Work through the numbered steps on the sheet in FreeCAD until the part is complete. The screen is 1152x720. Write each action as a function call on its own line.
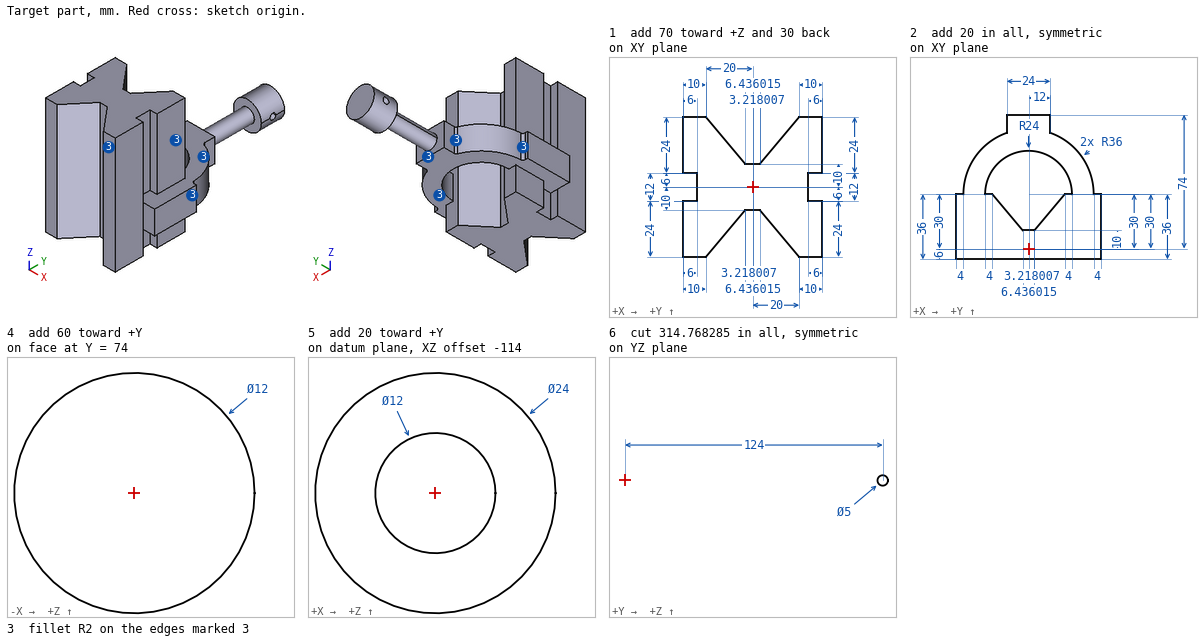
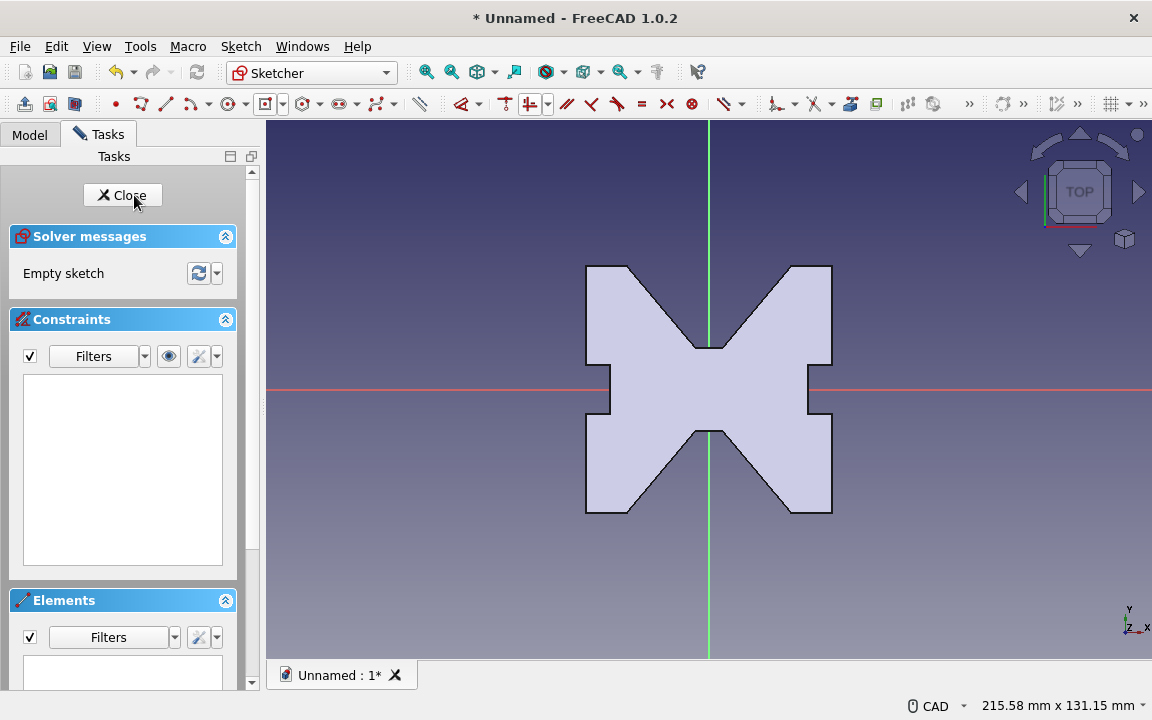
click(75, 104)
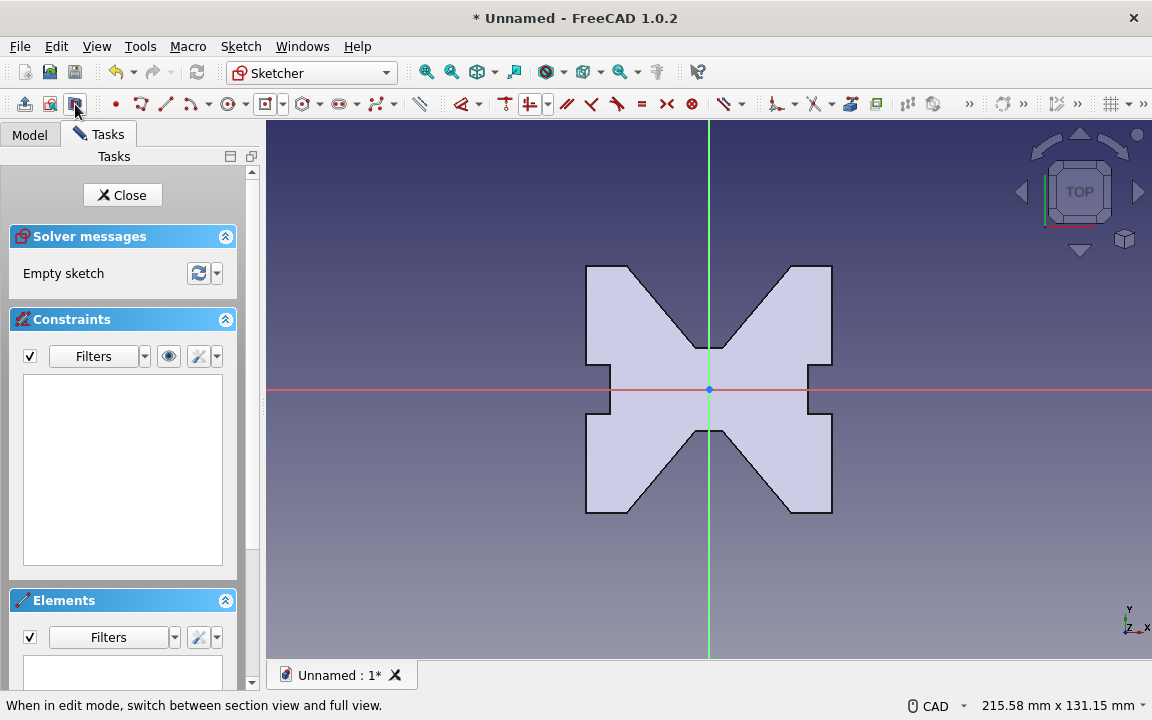
scroll(331, 631, down, 1)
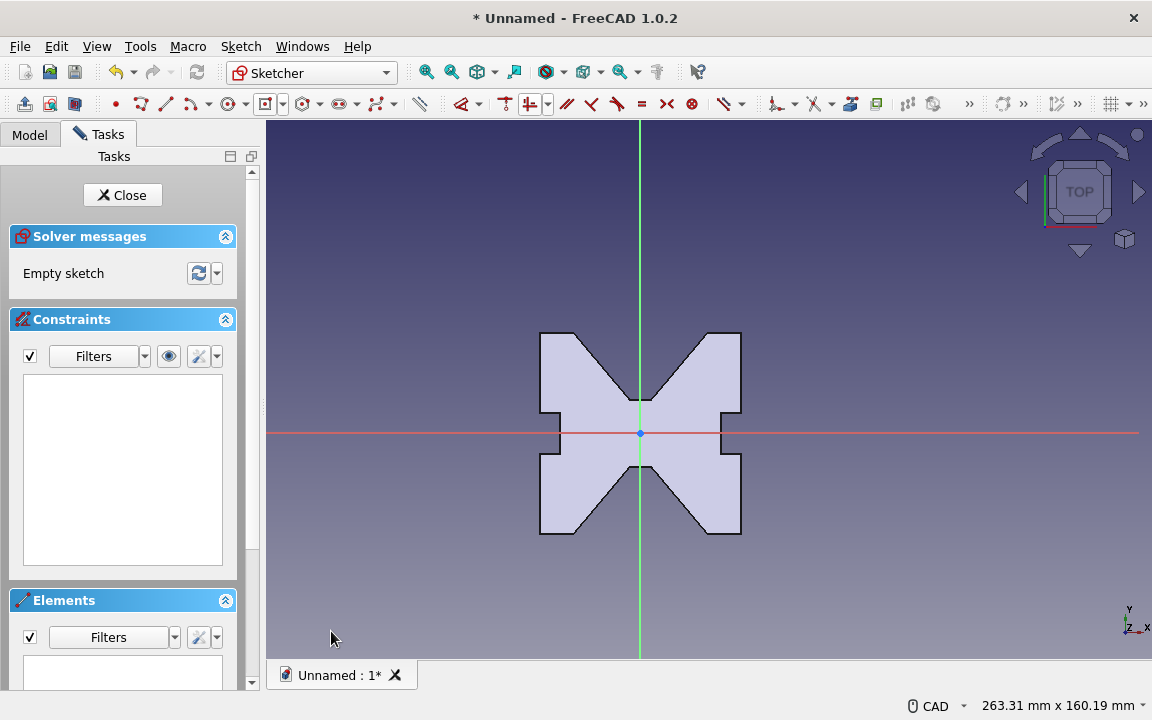
click(141, 104)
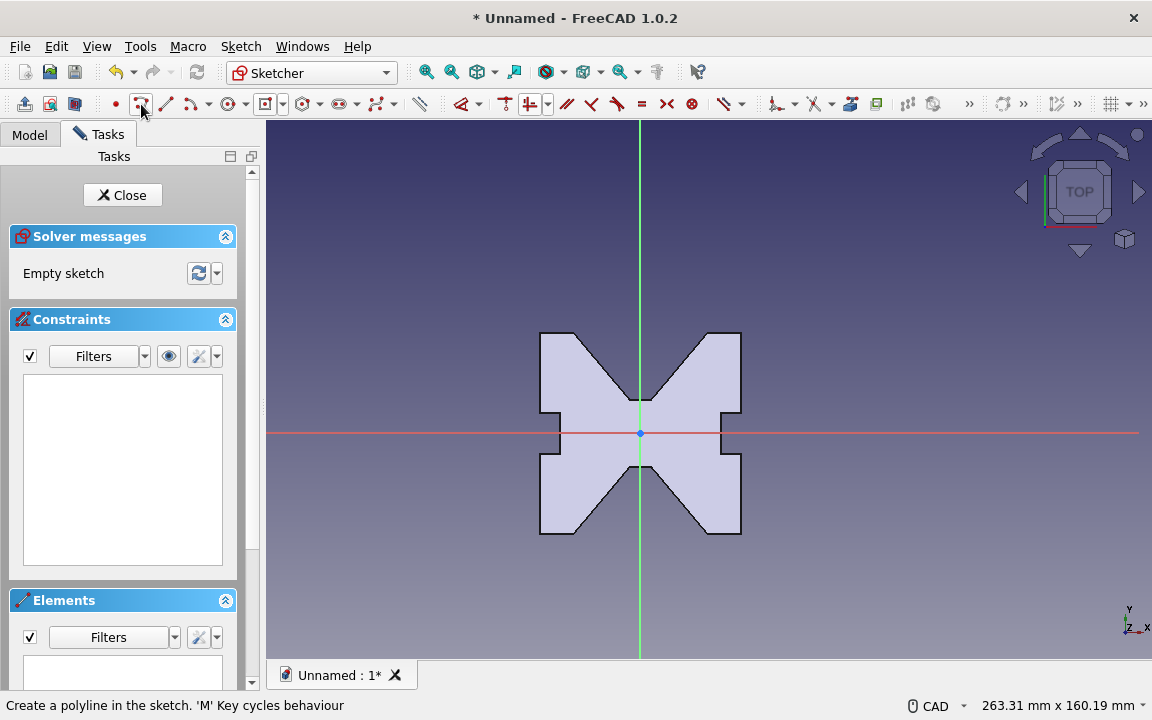
click(681, 218)
click(681, 184)
click(600, 184)
click(600, 218)
right_click(600, 218)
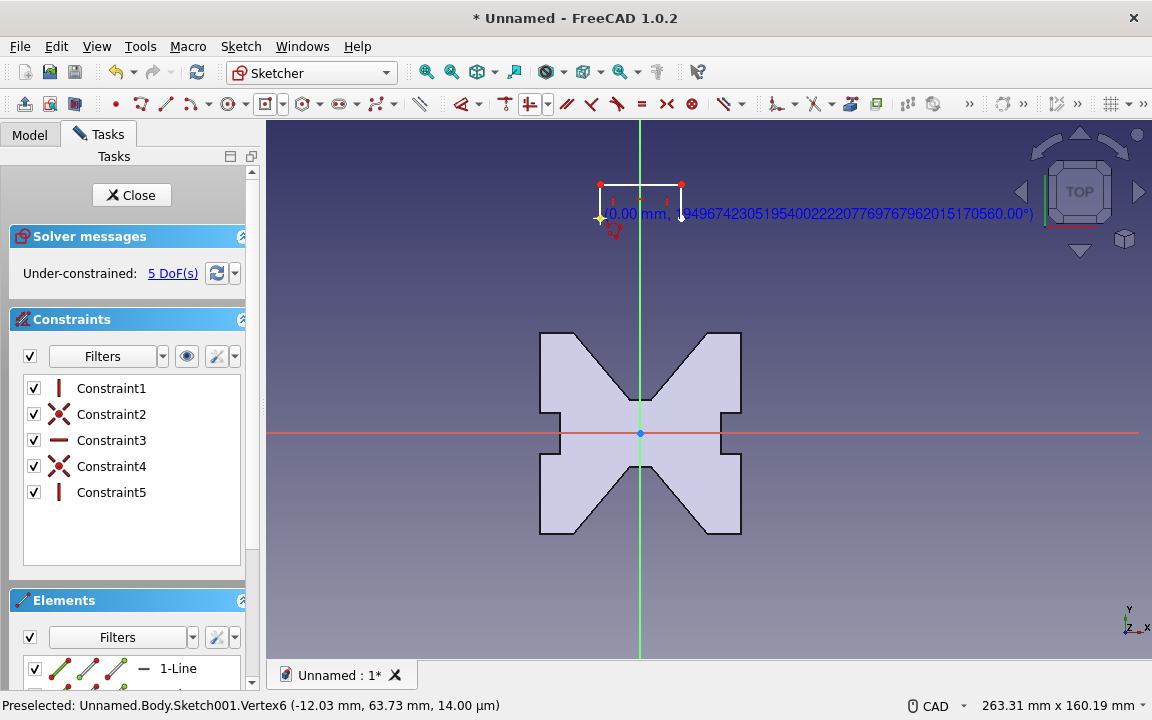
click(519, 333)
click(506, 333)
click(506, 454)
click(775, 454)
click(775, 333)
click(762, 333)
right_click(762, 333)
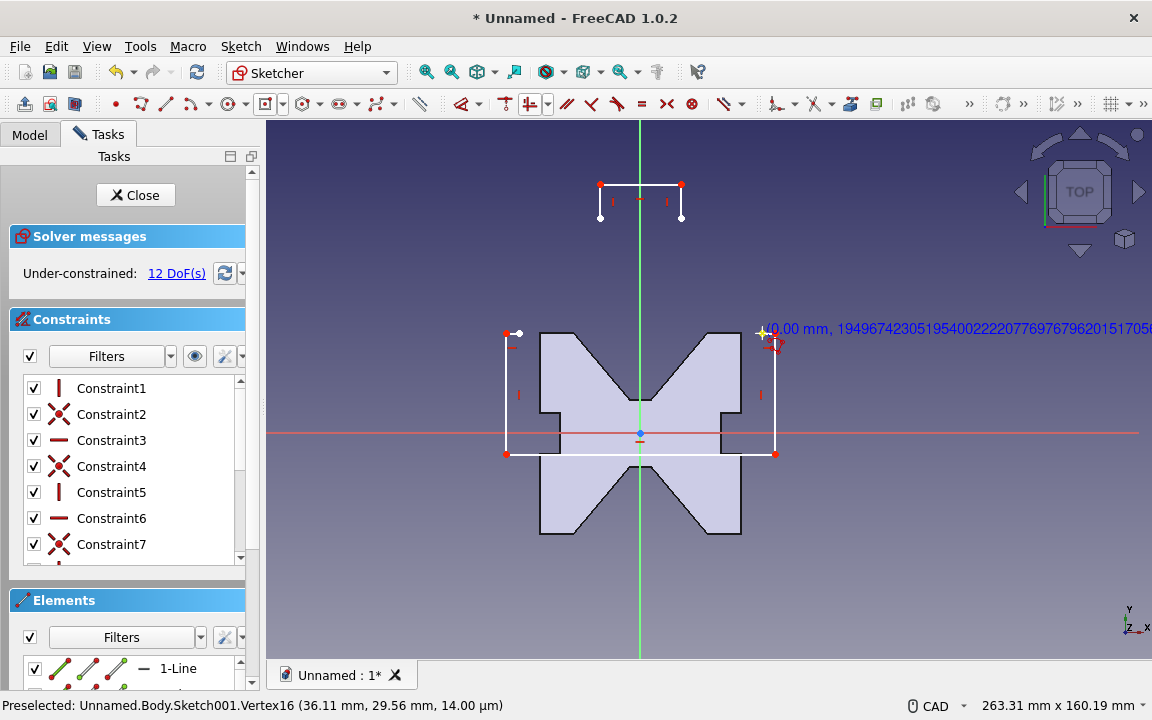
key(g)
key(3)
key(a)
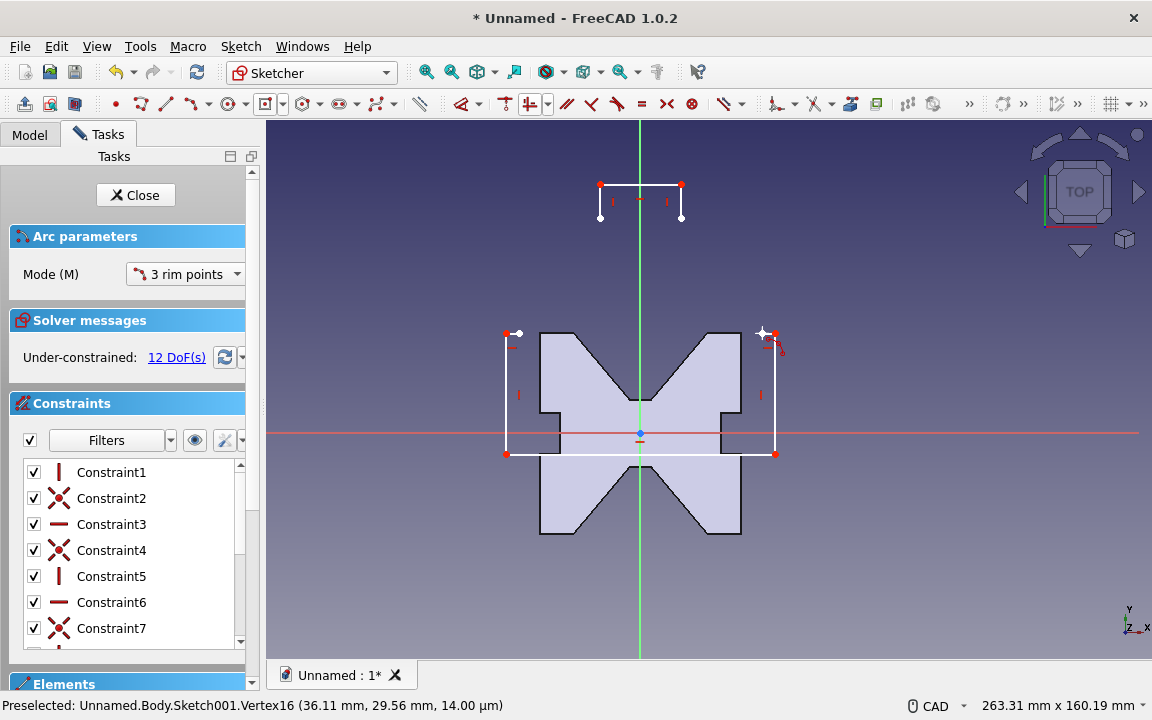
click(600, 219)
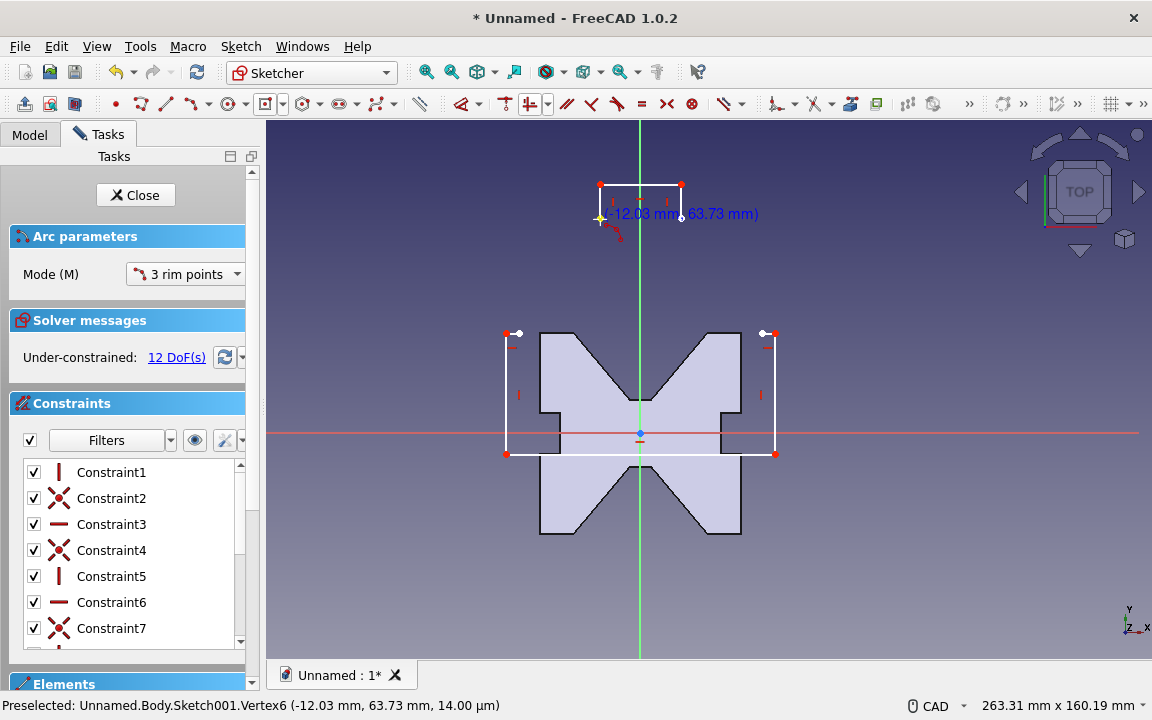
scroll(519, 333, up, 5)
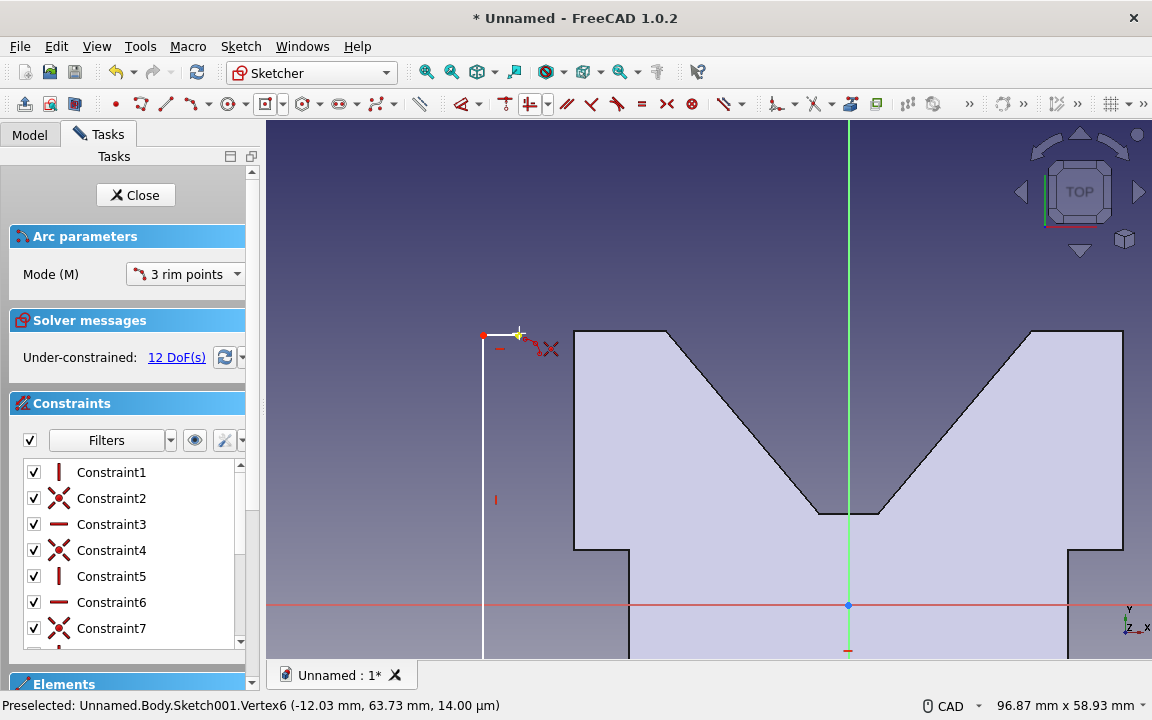
click(519, 335)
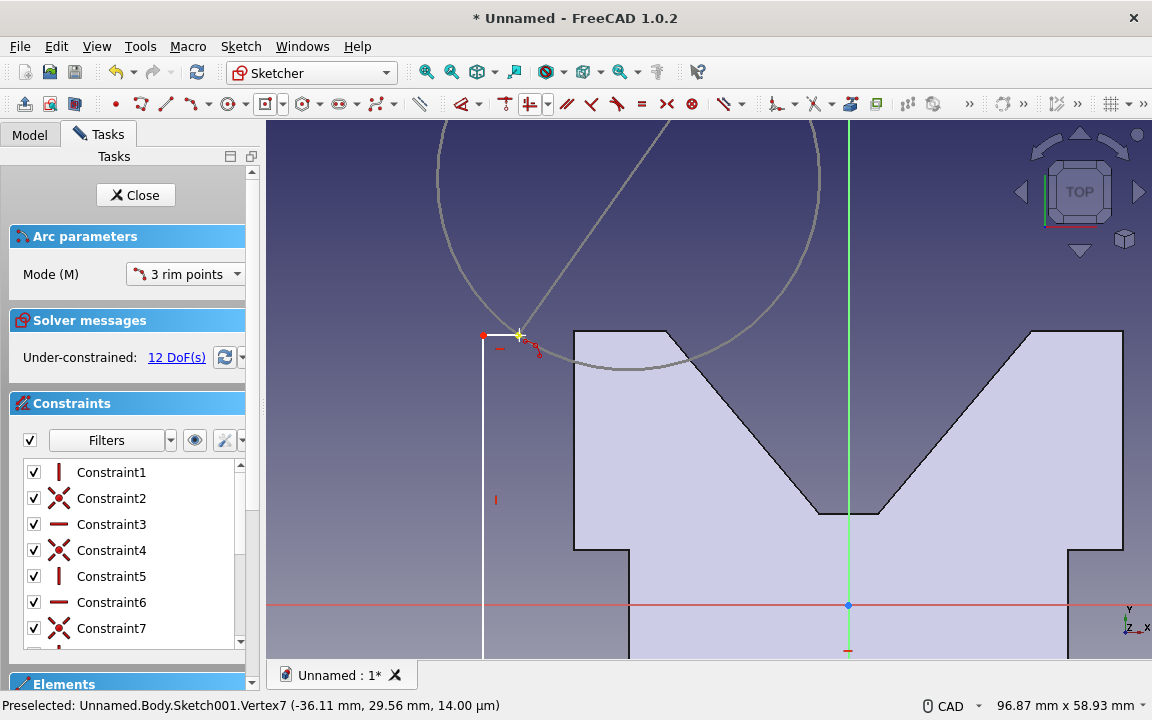
scroll(471, 467, down, 4)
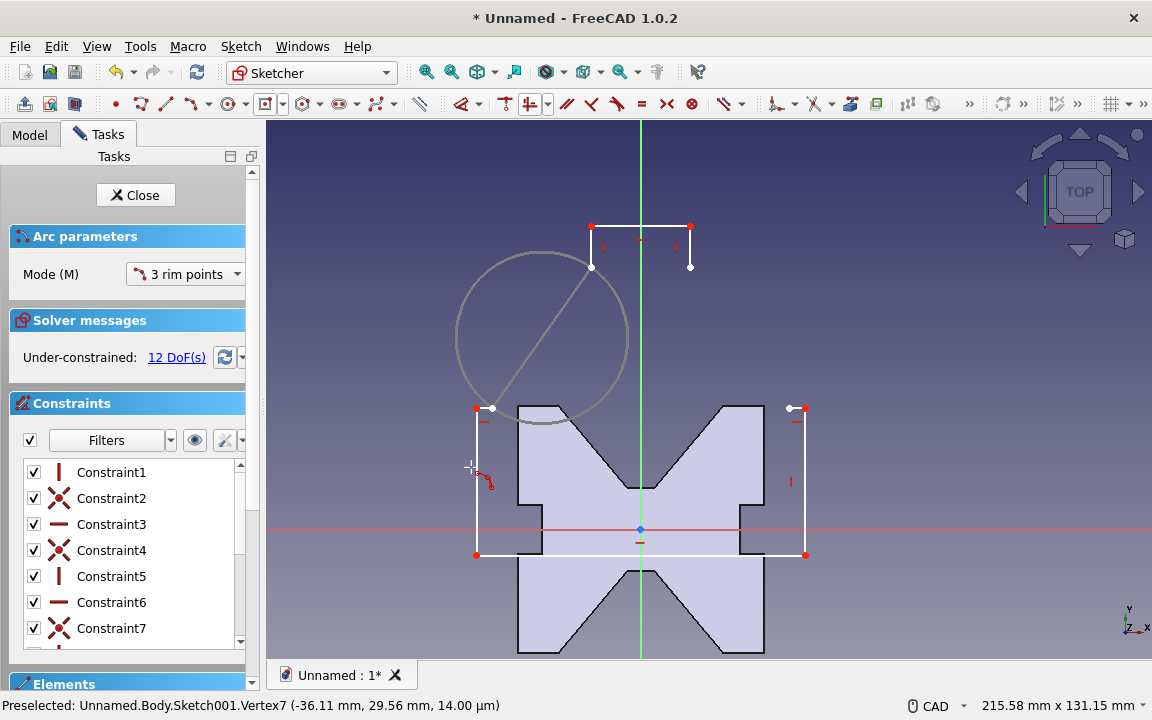
click(520, 321)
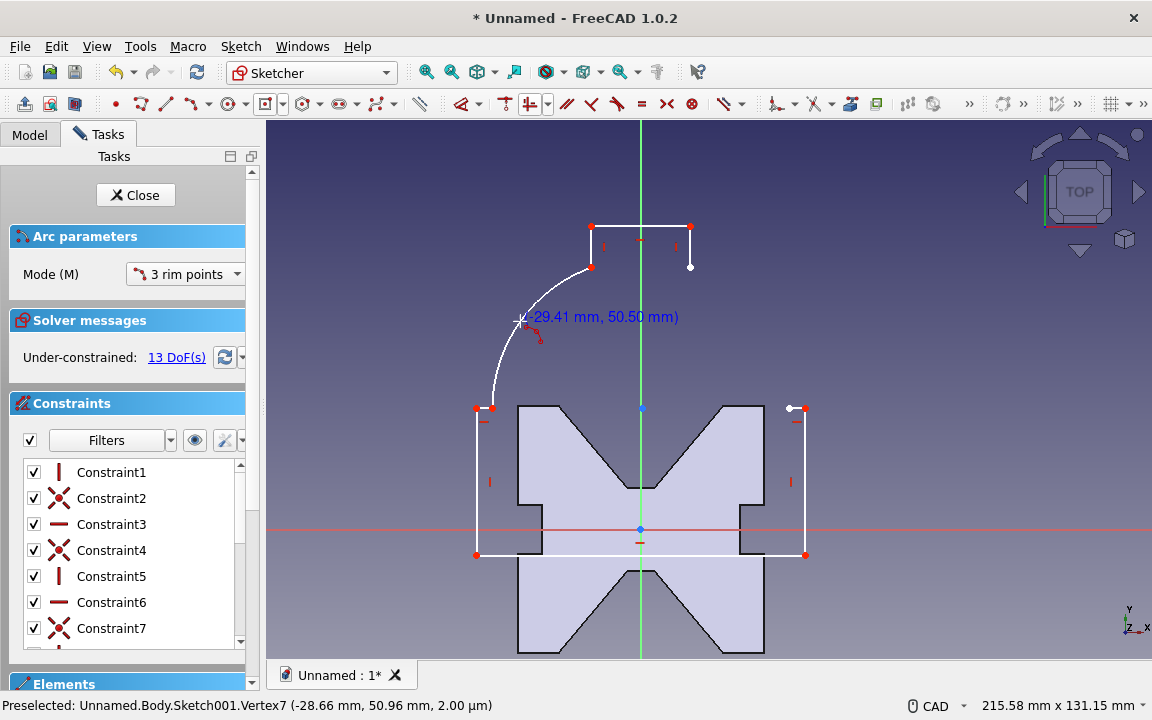
scroll(789, 406, up, 4)